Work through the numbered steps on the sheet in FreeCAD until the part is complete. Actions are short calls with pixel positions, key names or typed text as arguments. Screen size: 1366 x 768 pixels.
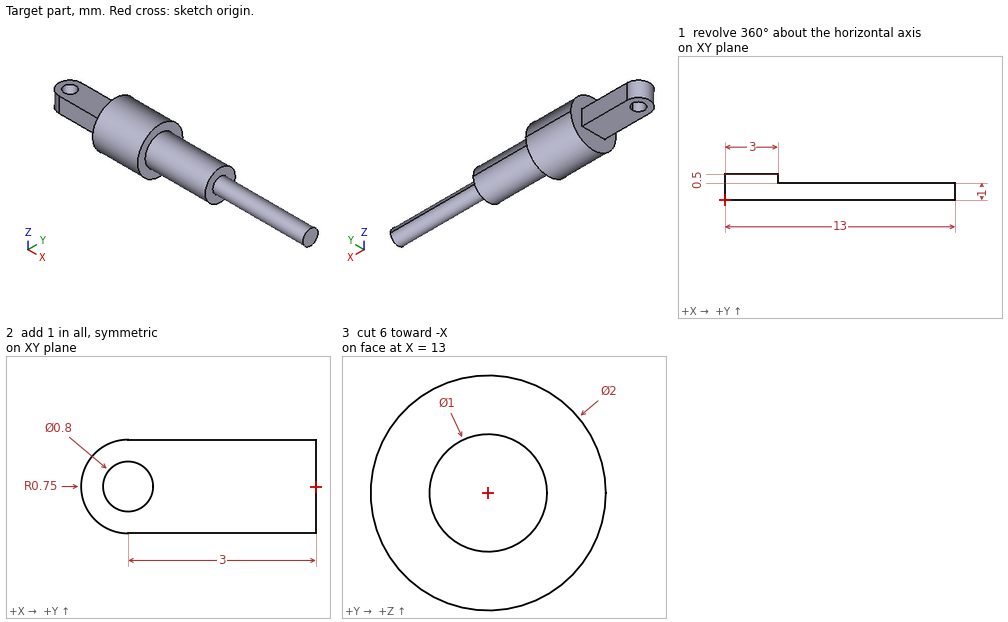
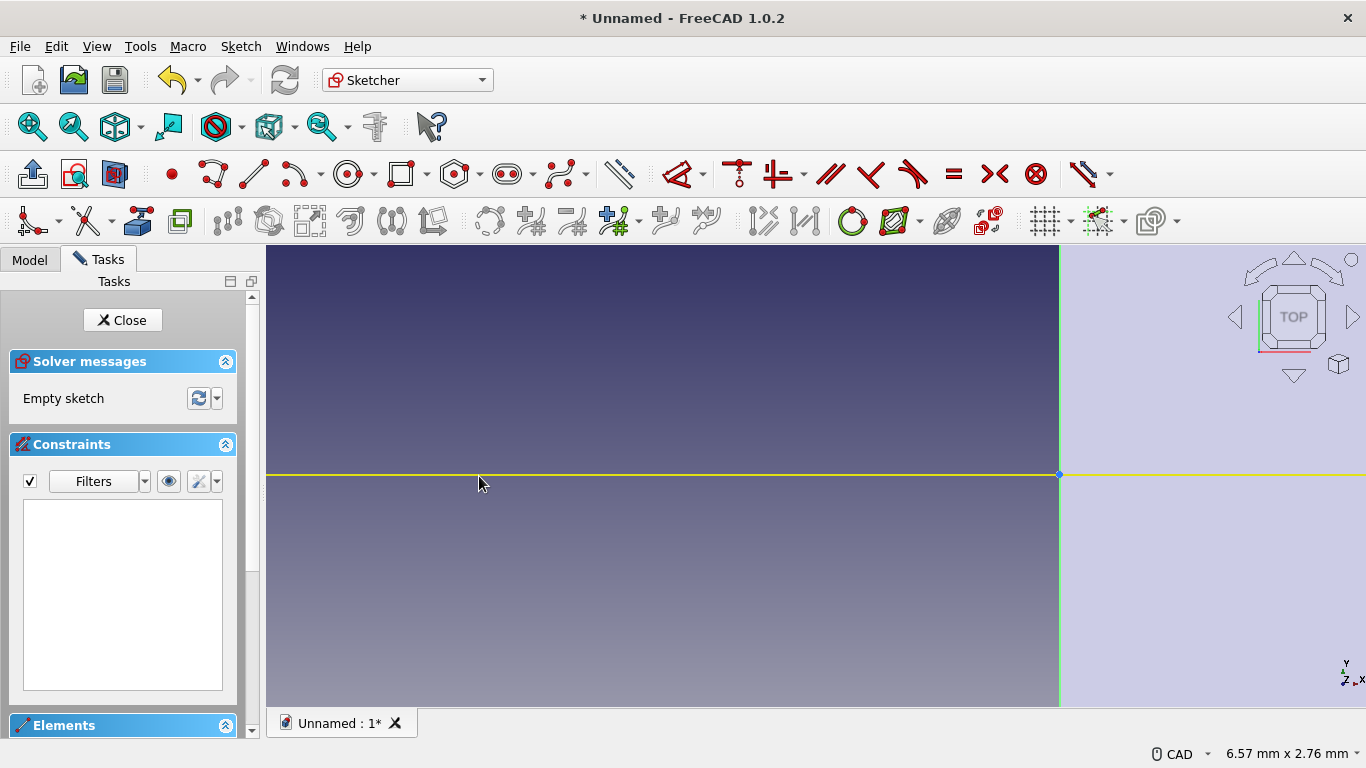
click(213, 174)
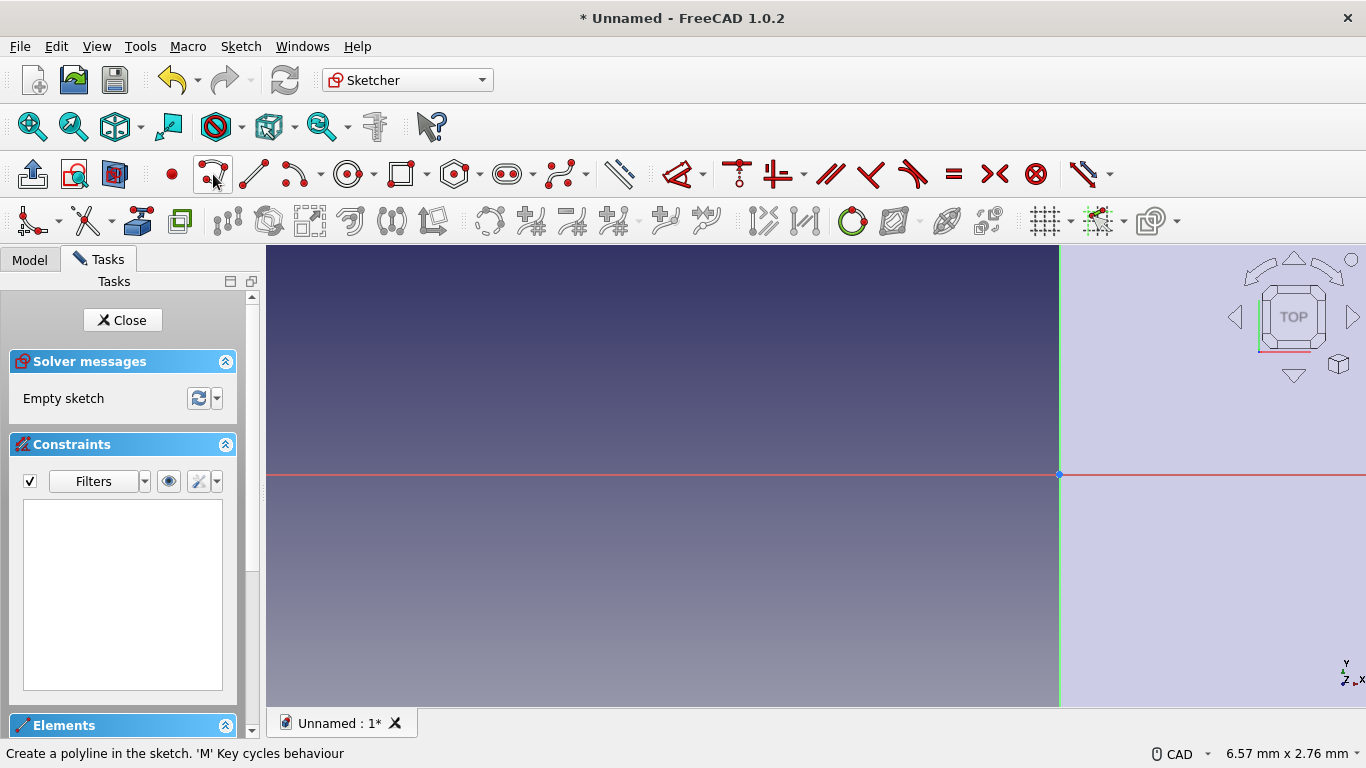
click(557, 600)
click(1060, 600)
click(1051, 349)
click(557, 349)
right_click(557, 349)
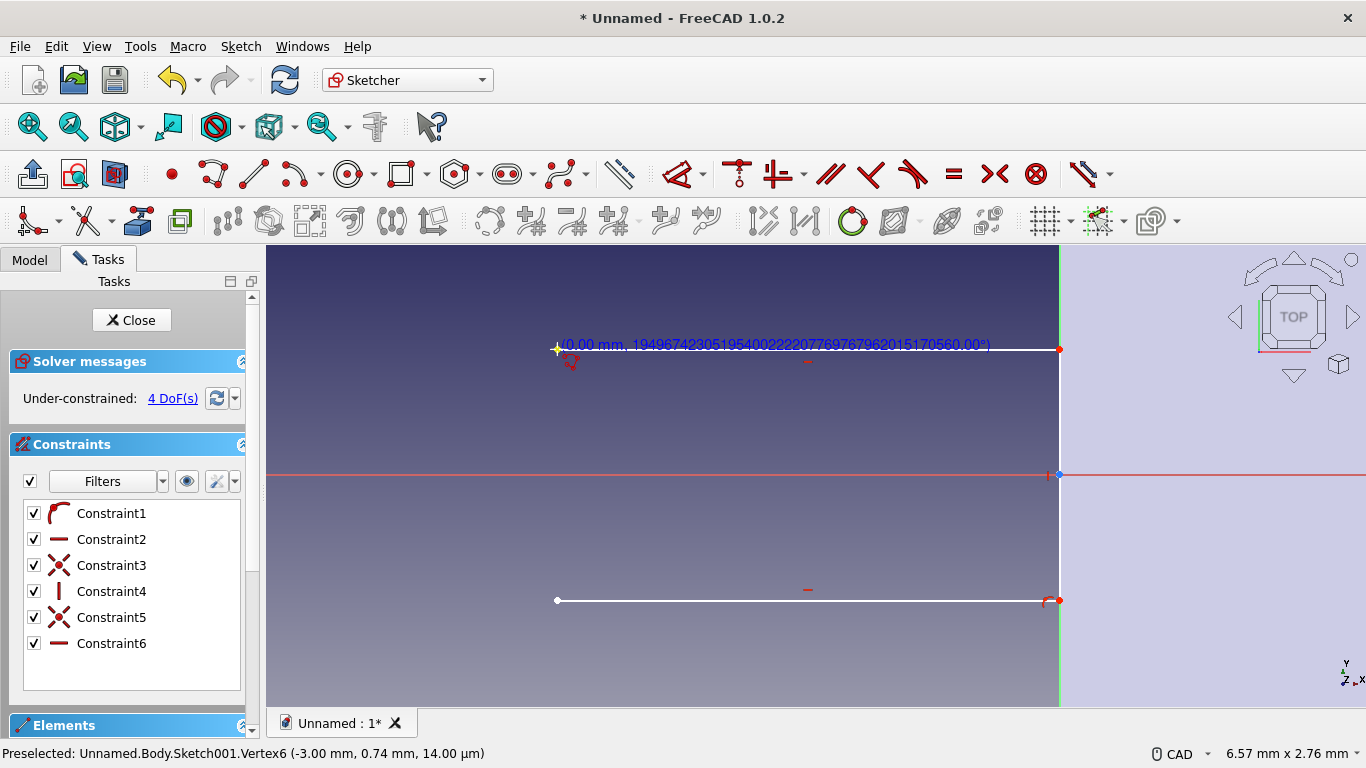
key(g)
key(3)
key(a)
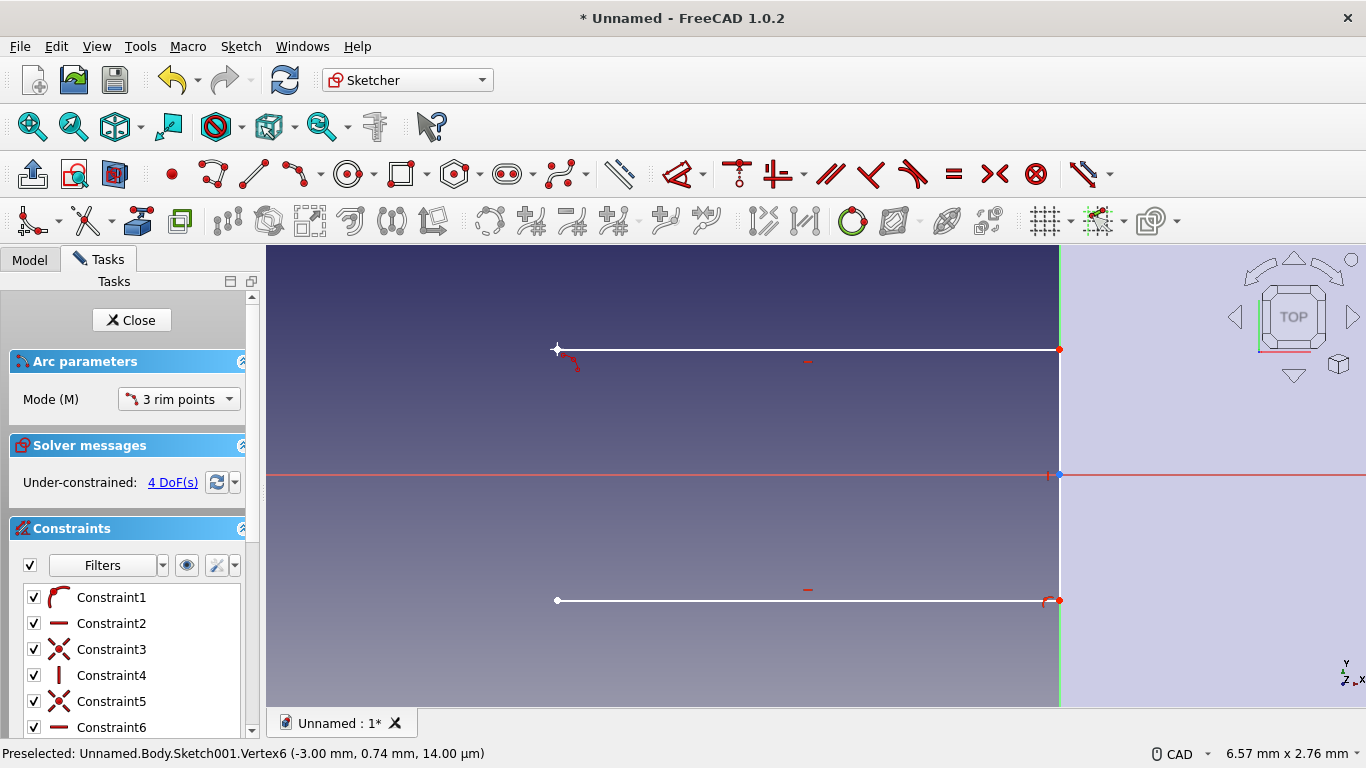
click(557, 350)
click(557, 601)
click(438, 436)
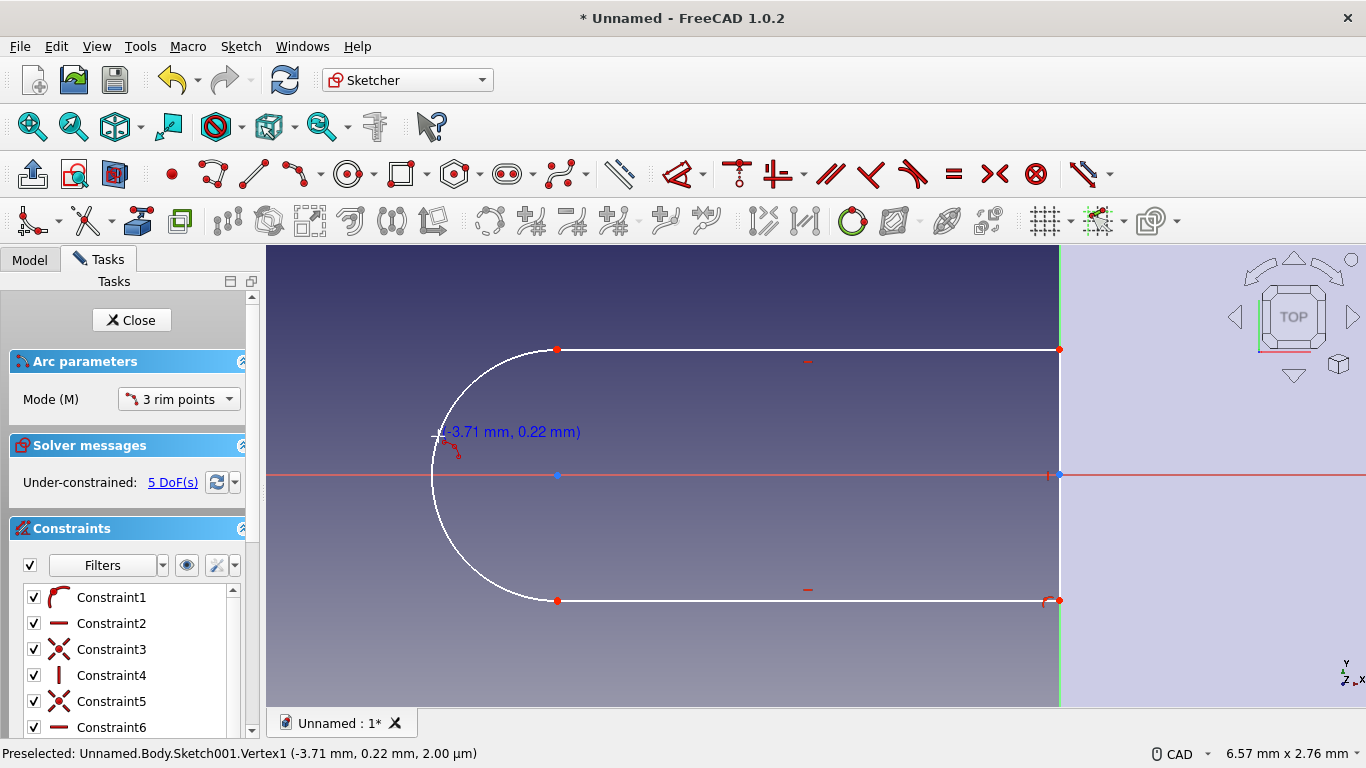
key(g)
key(c)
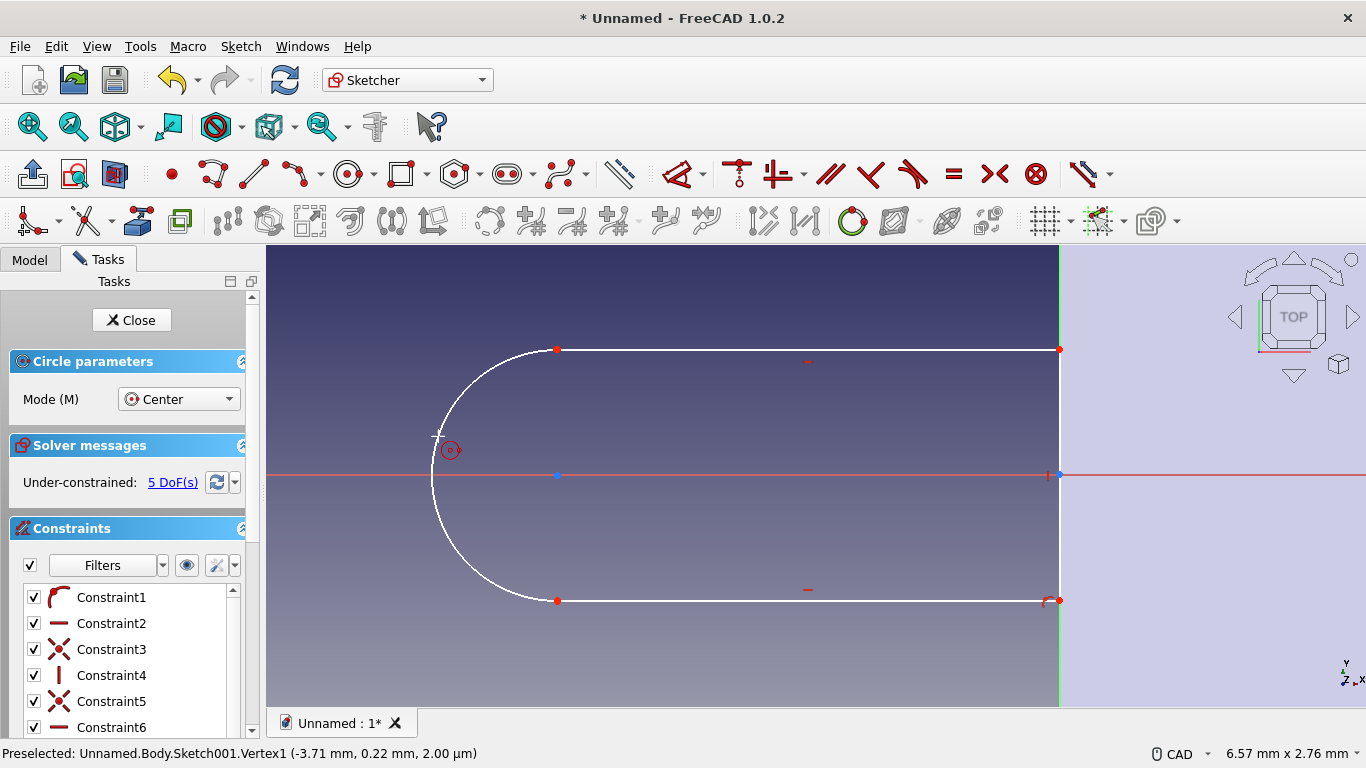
click(557, 475)
click(605, 427)
key(Escape)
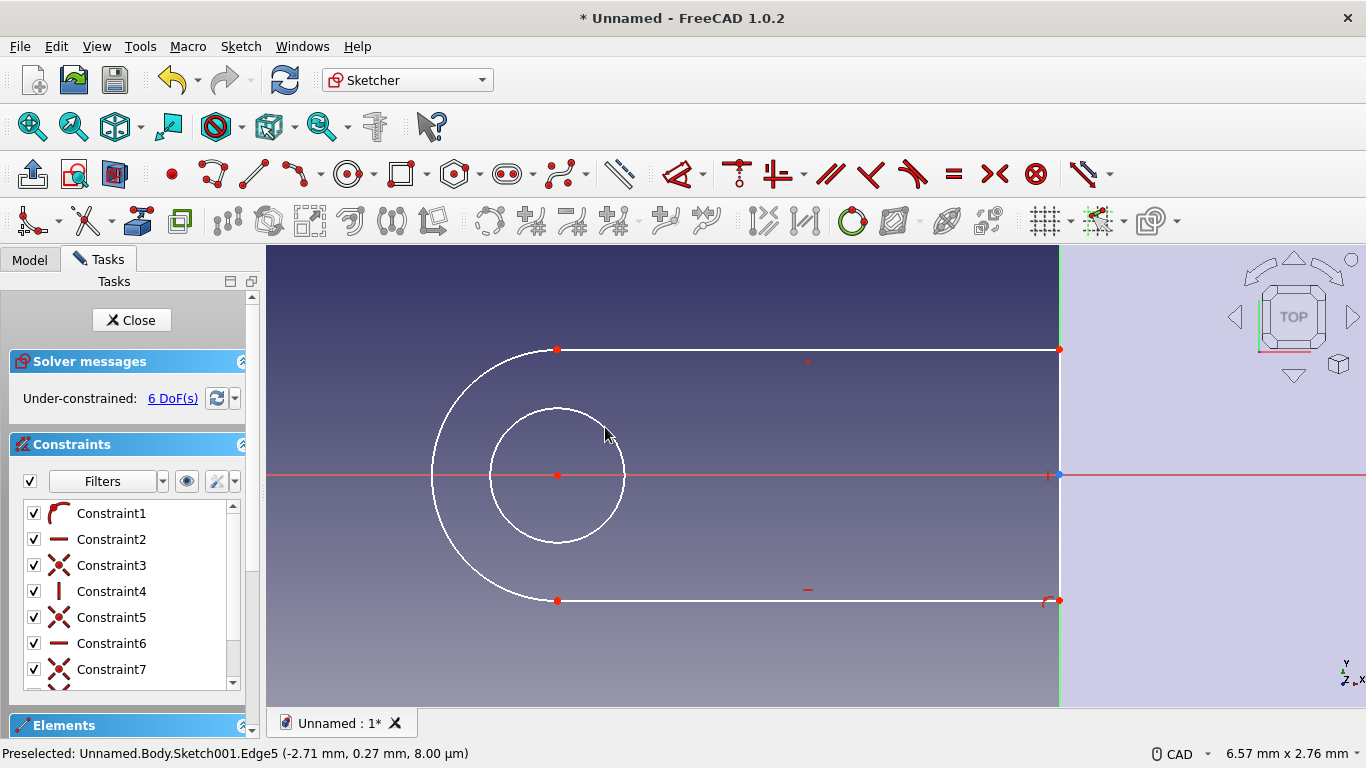
click(708, 601)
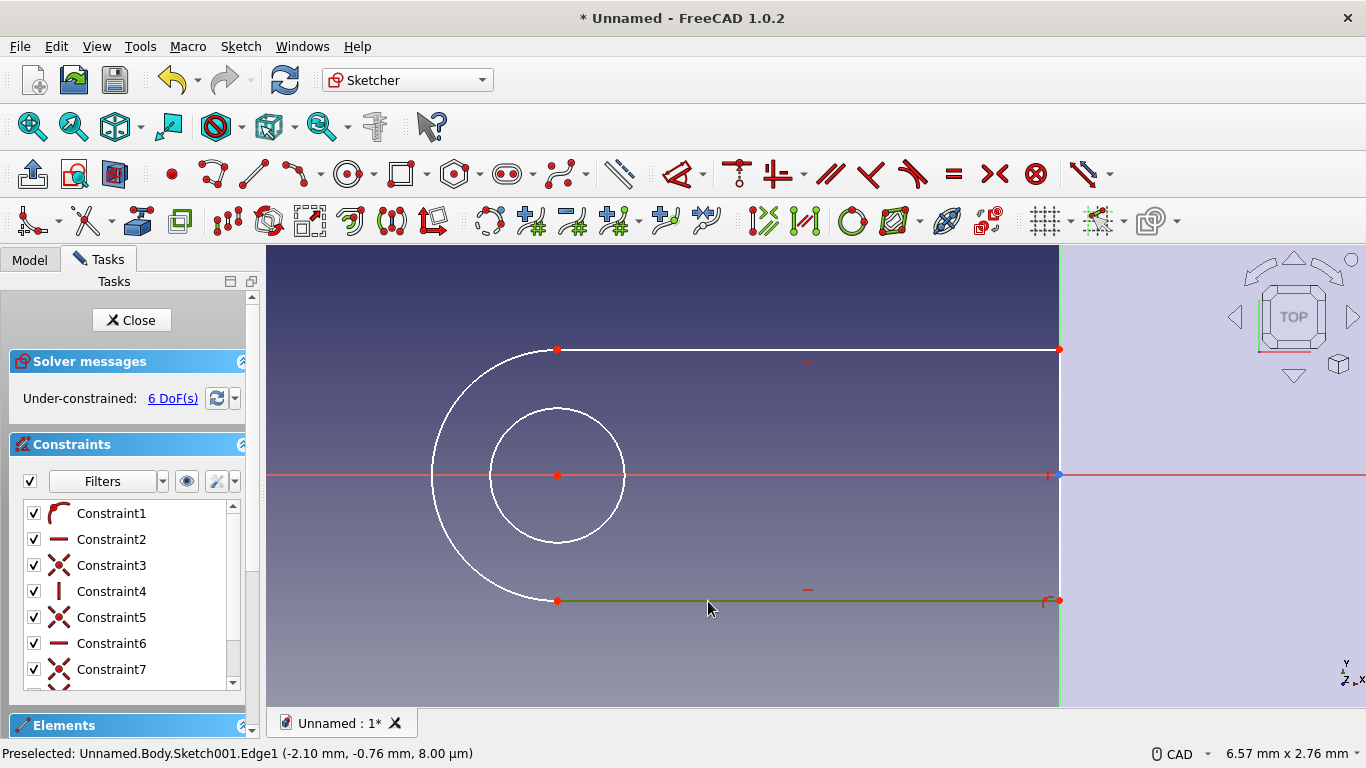
click(456, 402)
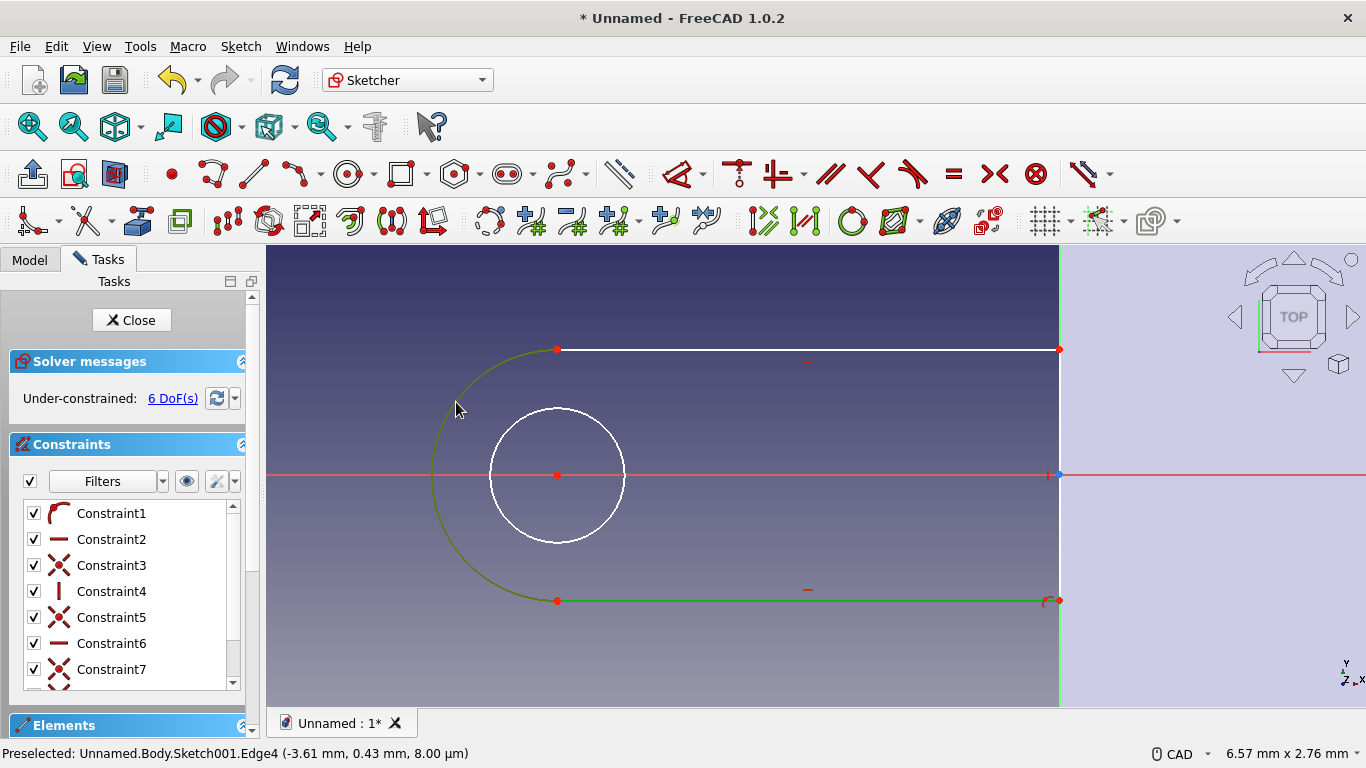
click(913, 174)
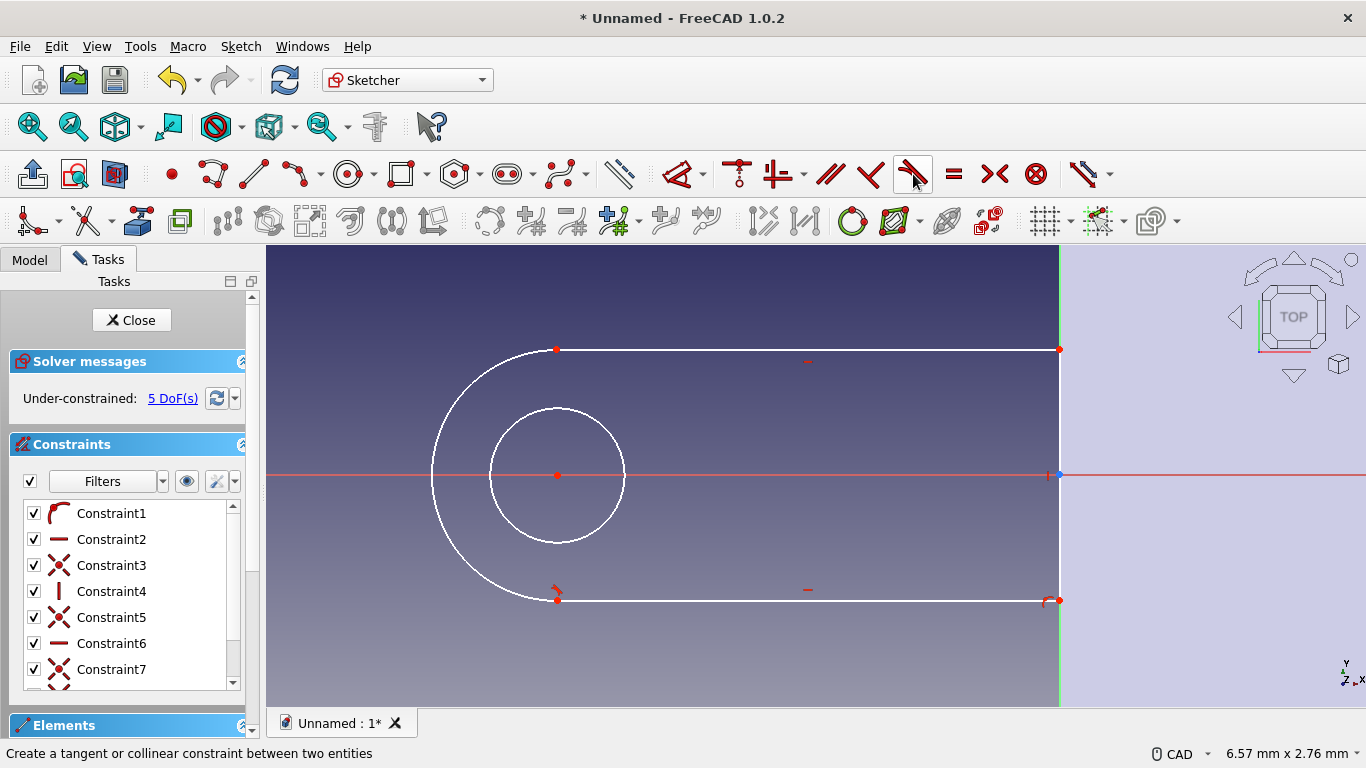
click(909, 350)